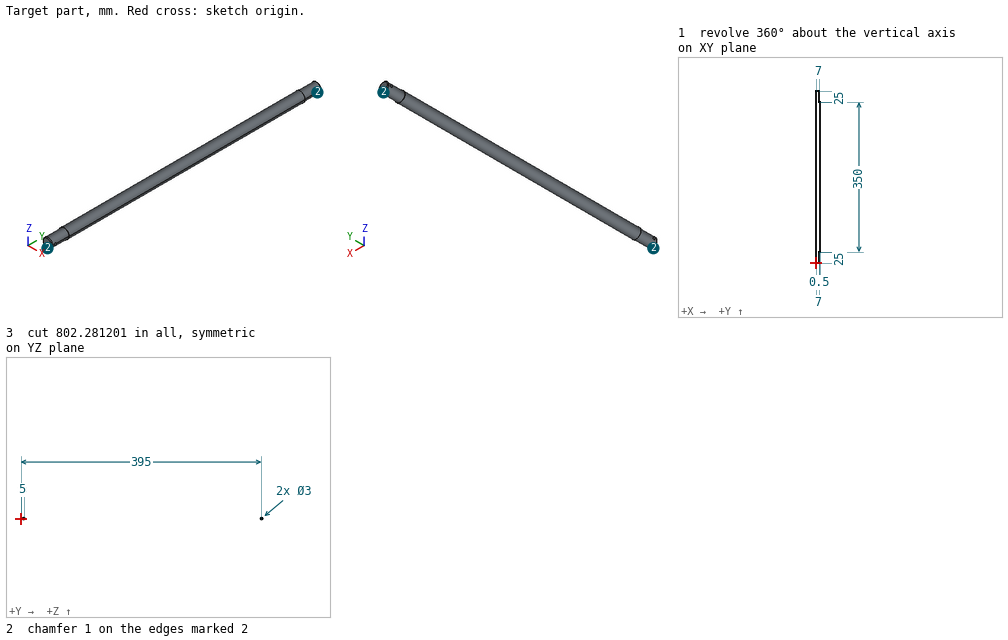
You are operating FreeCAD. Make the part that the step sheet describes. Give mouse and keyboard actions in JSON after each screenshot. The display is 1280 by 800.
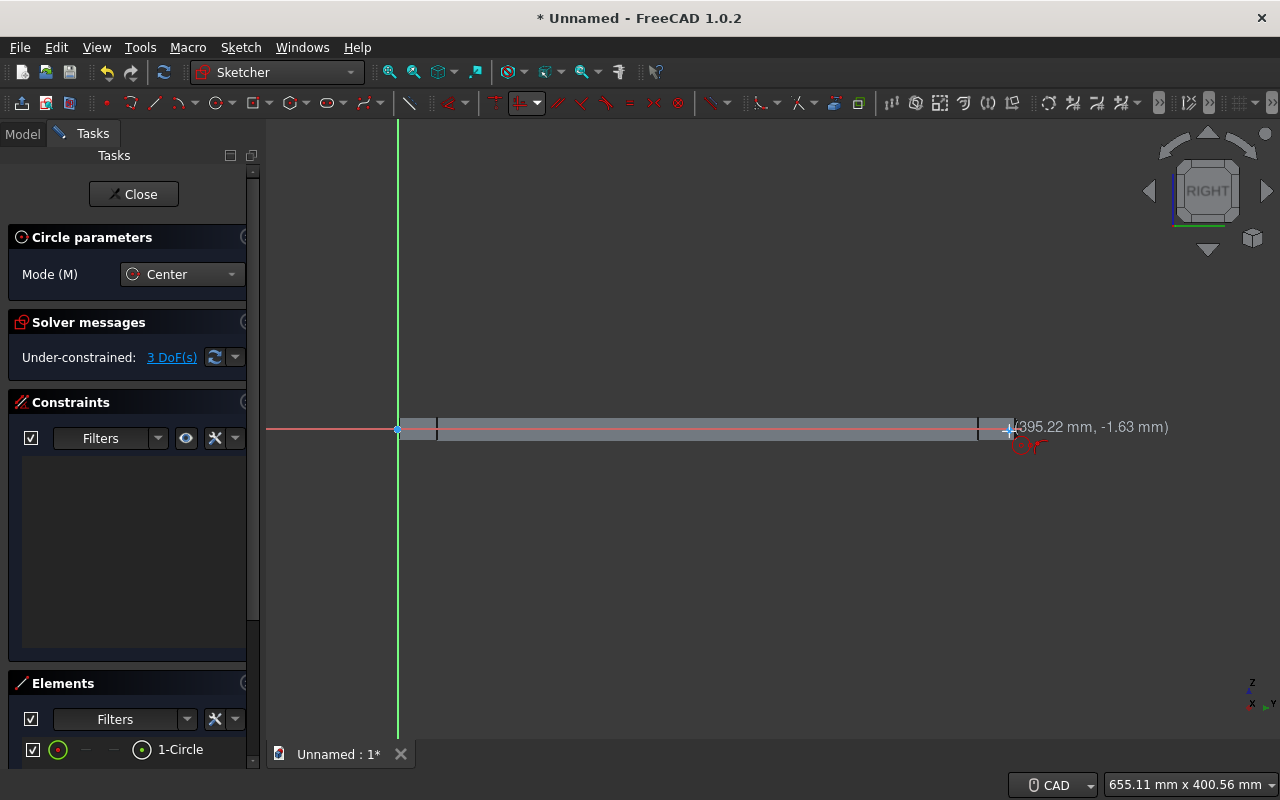
{"action": "scroll", "coordinate": [406, 429], "scroll_direction": "up", "scroll_amount": 12}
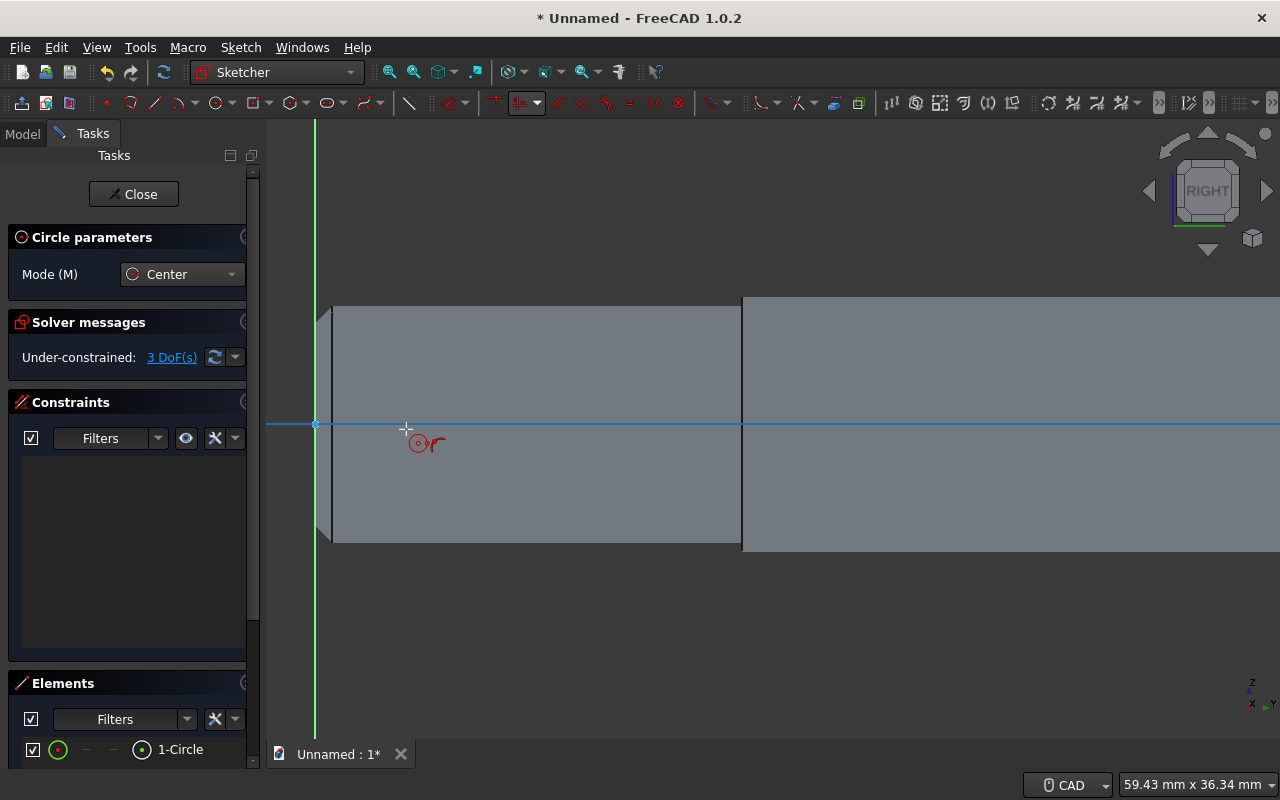
{"action": "scroll", "coordinate": [406, 429], "scroll_direction": "down", "scroll_amount": 12}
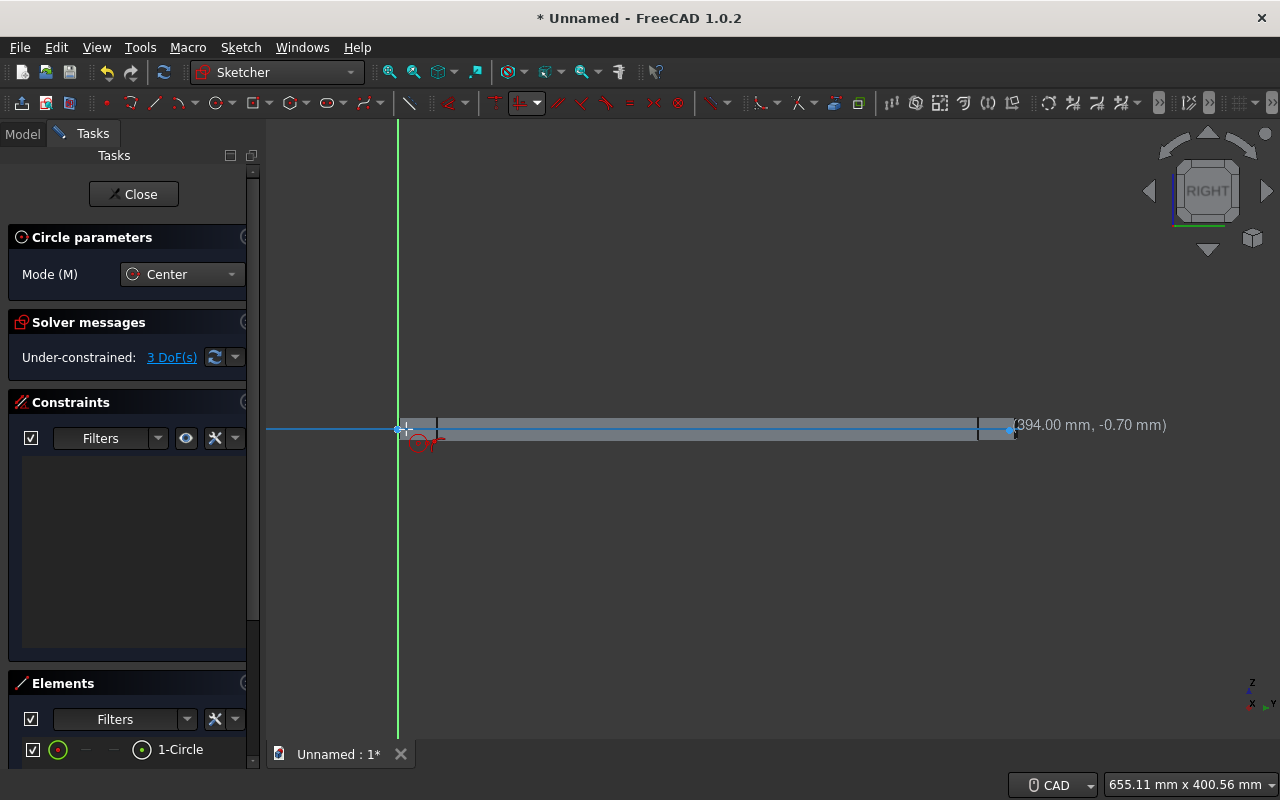
{"action": "scroll", "coordinate": [406, 429], "scroll_direction": "up", "scroll_amount": 4}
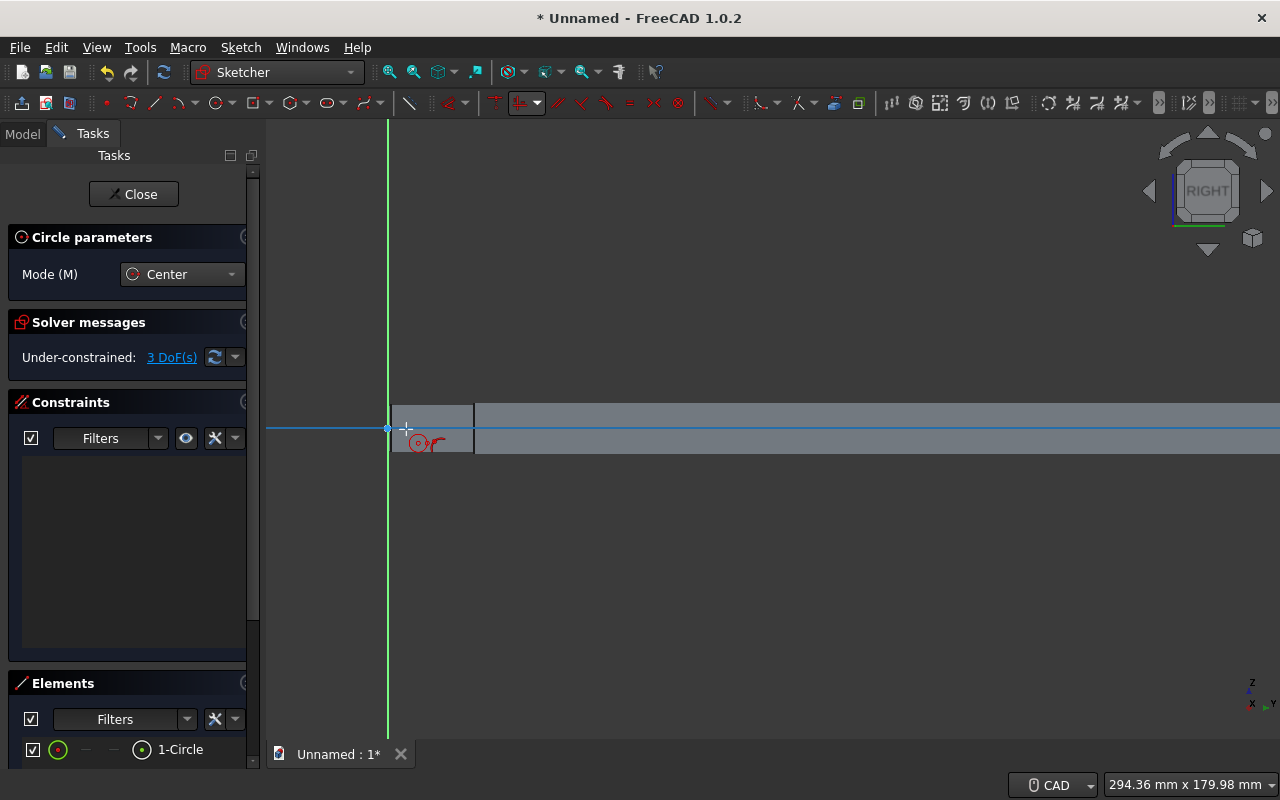
{"action": "left_click", "coordinate": [405, 428]}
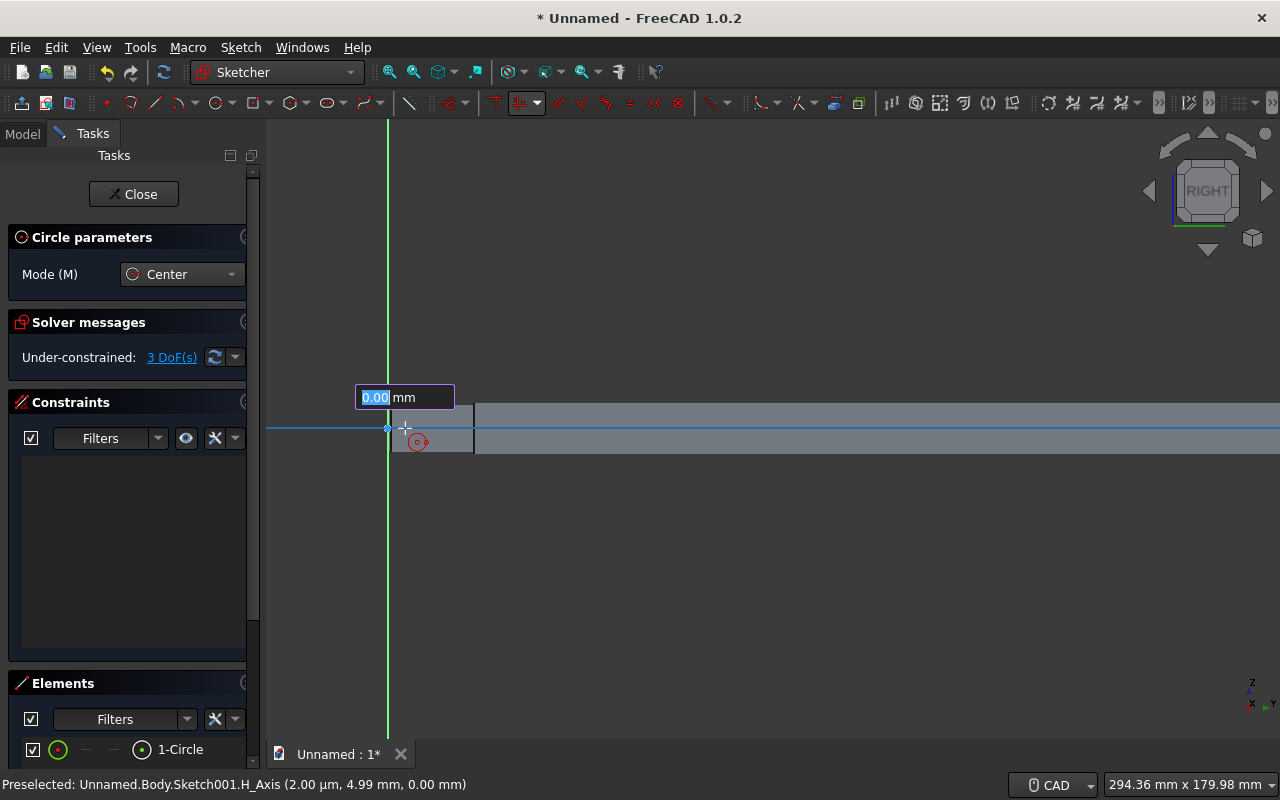
{"action": "scroll", "coordinate": [407, 424], "scroll_direction": "up", "scroll_amount": 6}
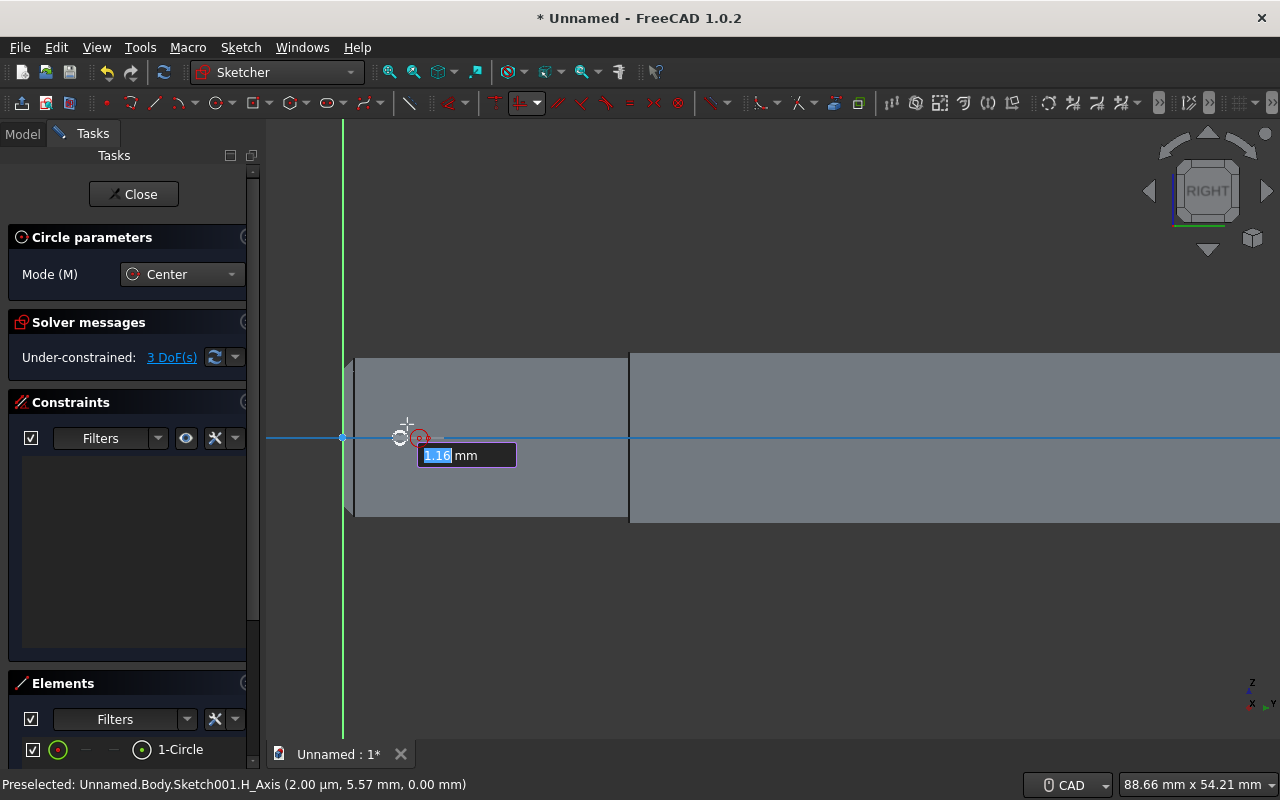
{"action": "left_click", "coordinate": [406, 422]}
{"action": "key", "text": "Escape"}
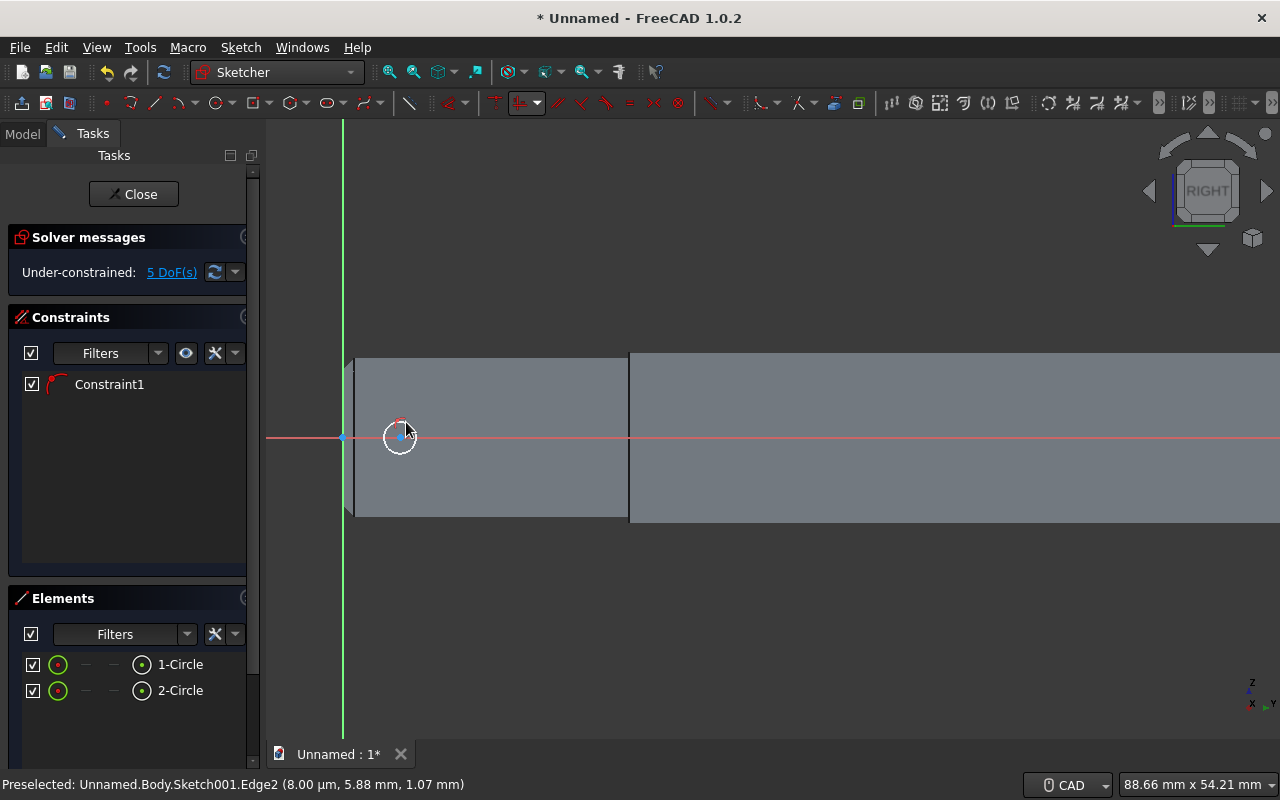
{"action": "scroll", "coordinate": [406, 428], "scroll_direction": "down", "scroll_amount": 10}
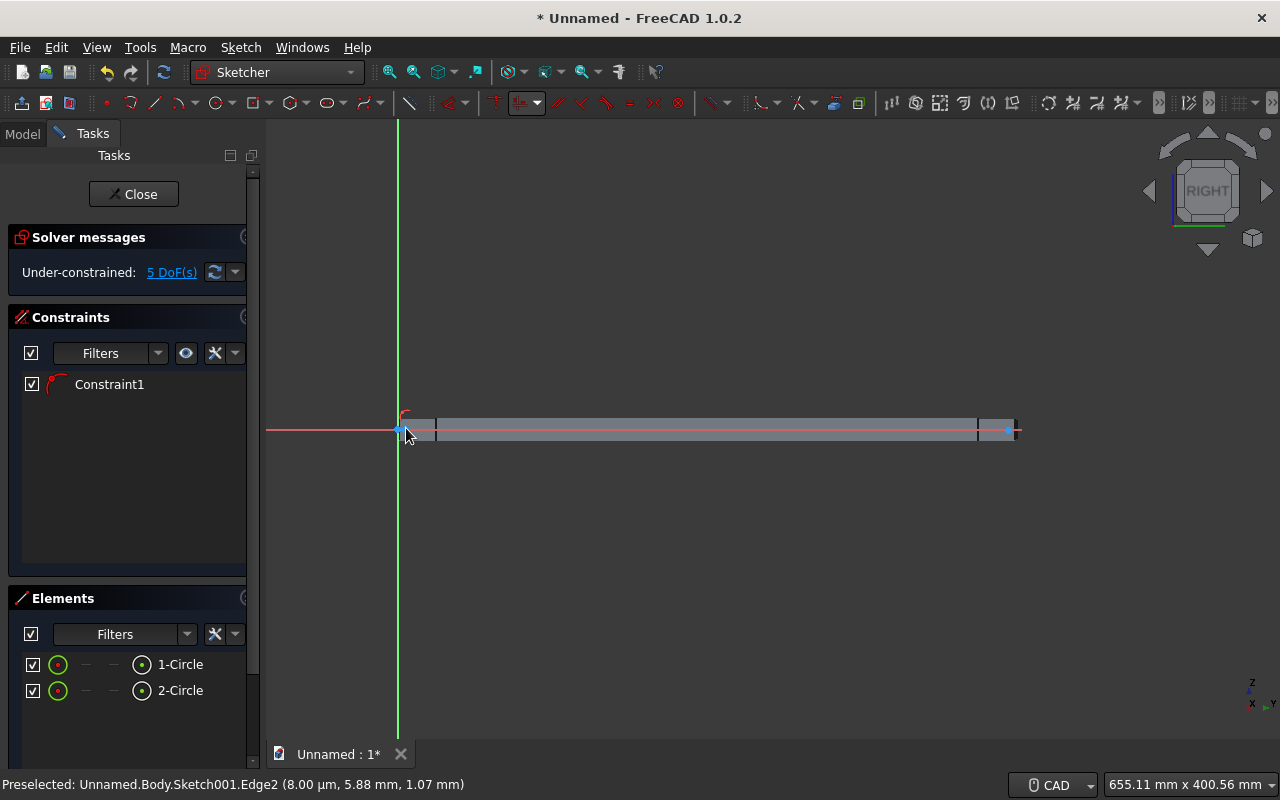
{"action": "scroll", "coordinate": [1010, 430], "scroll_direction": "up", "scroll_amount": 13}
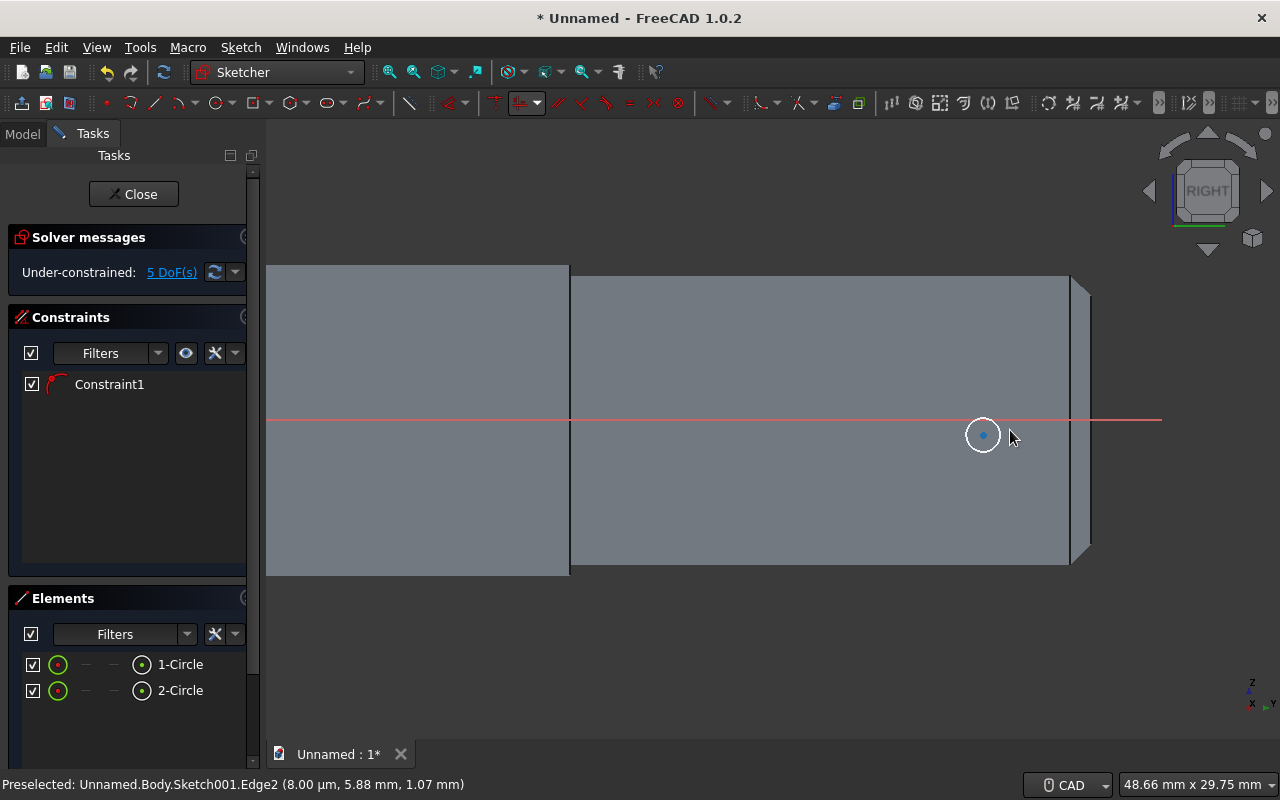
{"action": "left_click", "coordinate": [995, 423]}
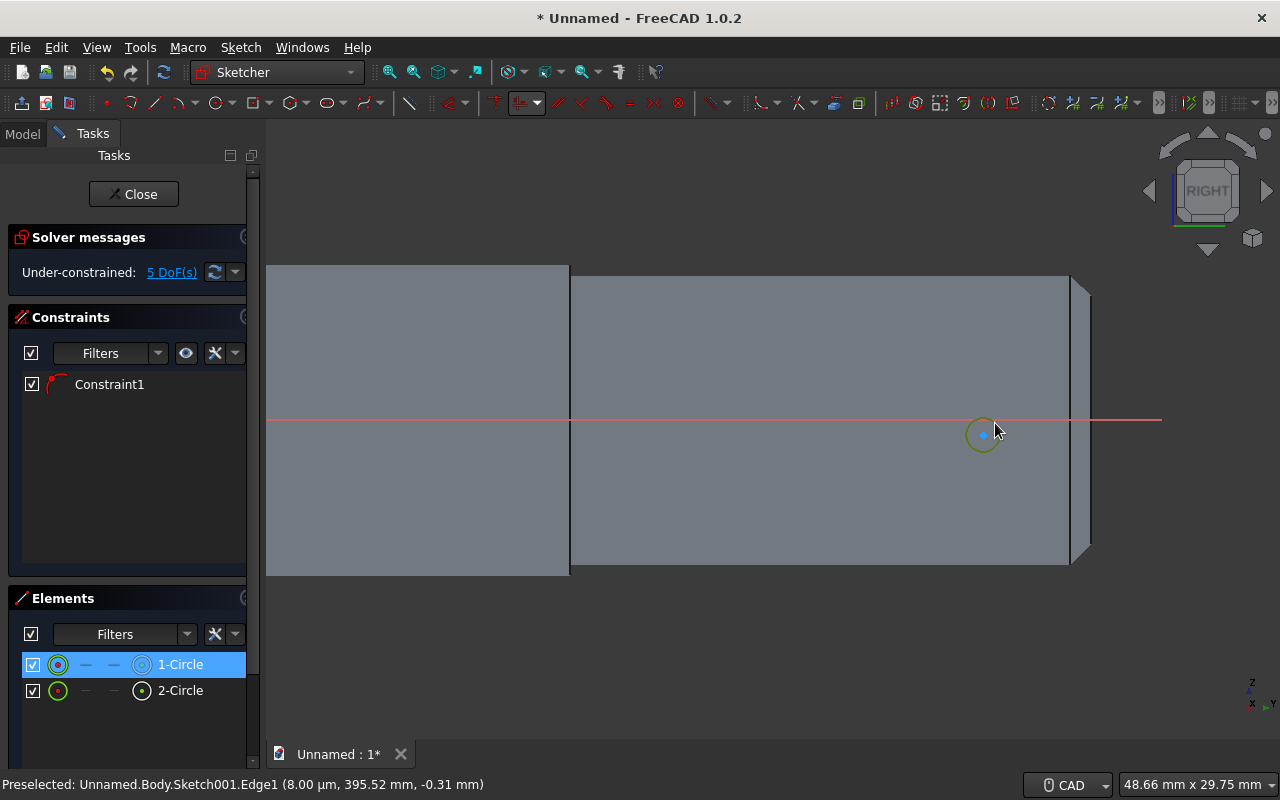
{"action": "scroll", "coordinate": [1011, 430], "scroll_direction": "down", "scroll_amount": 13}